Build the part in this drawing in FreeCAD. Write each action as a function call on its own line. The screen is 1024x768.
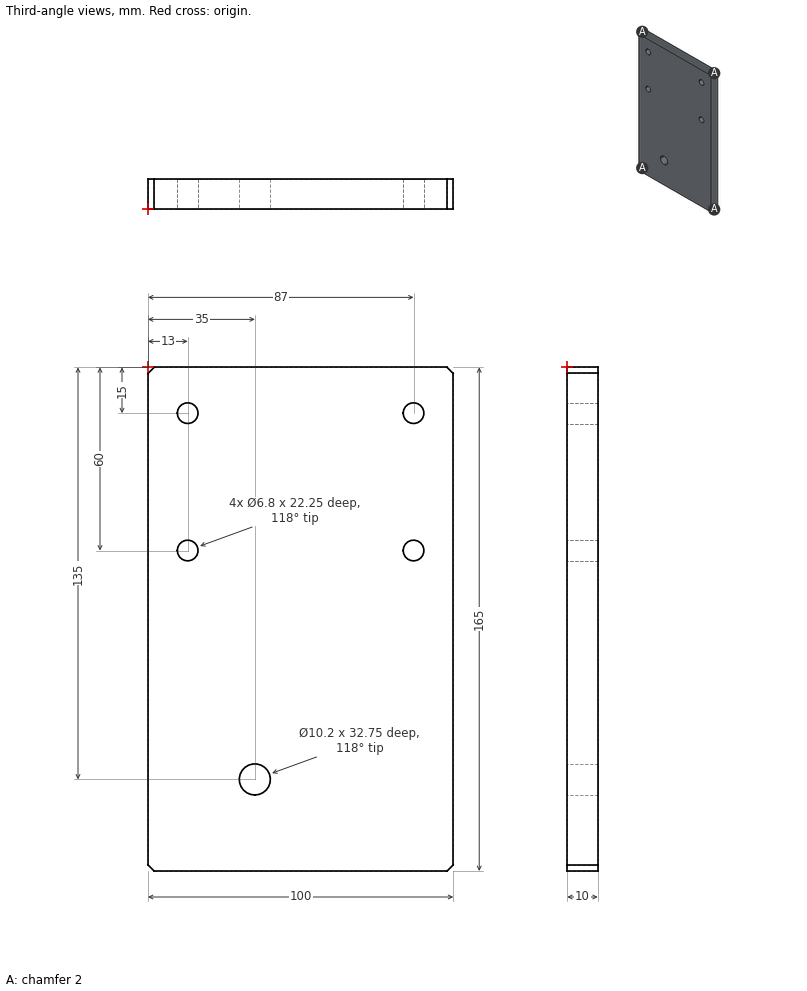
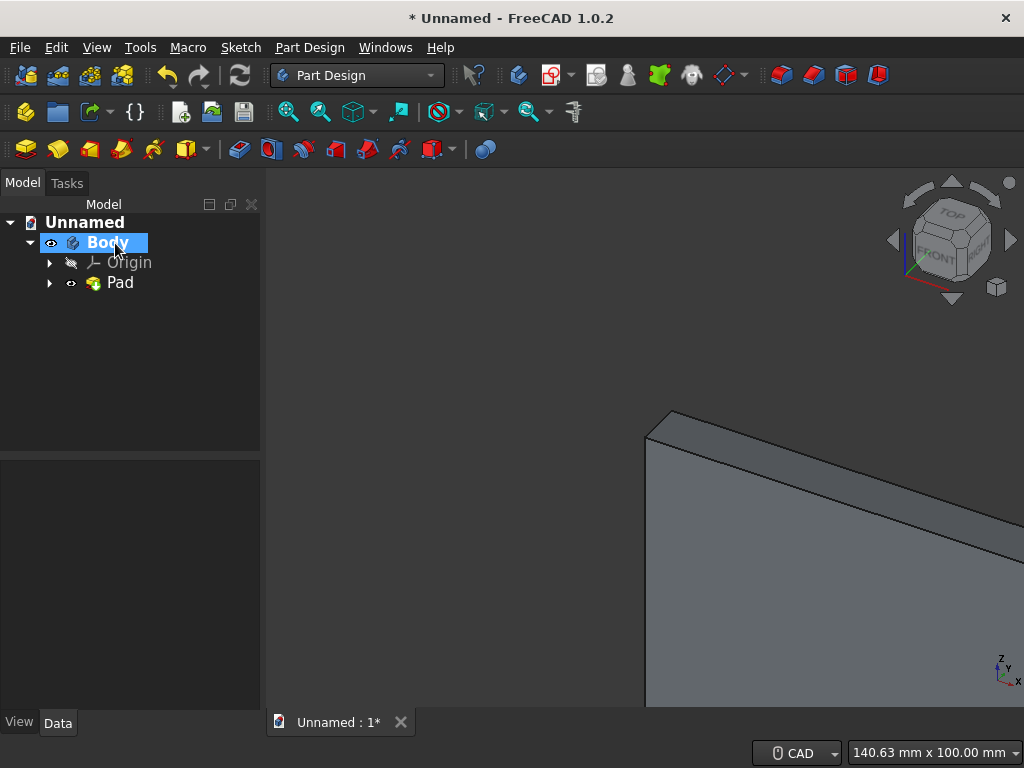
click(290, 112)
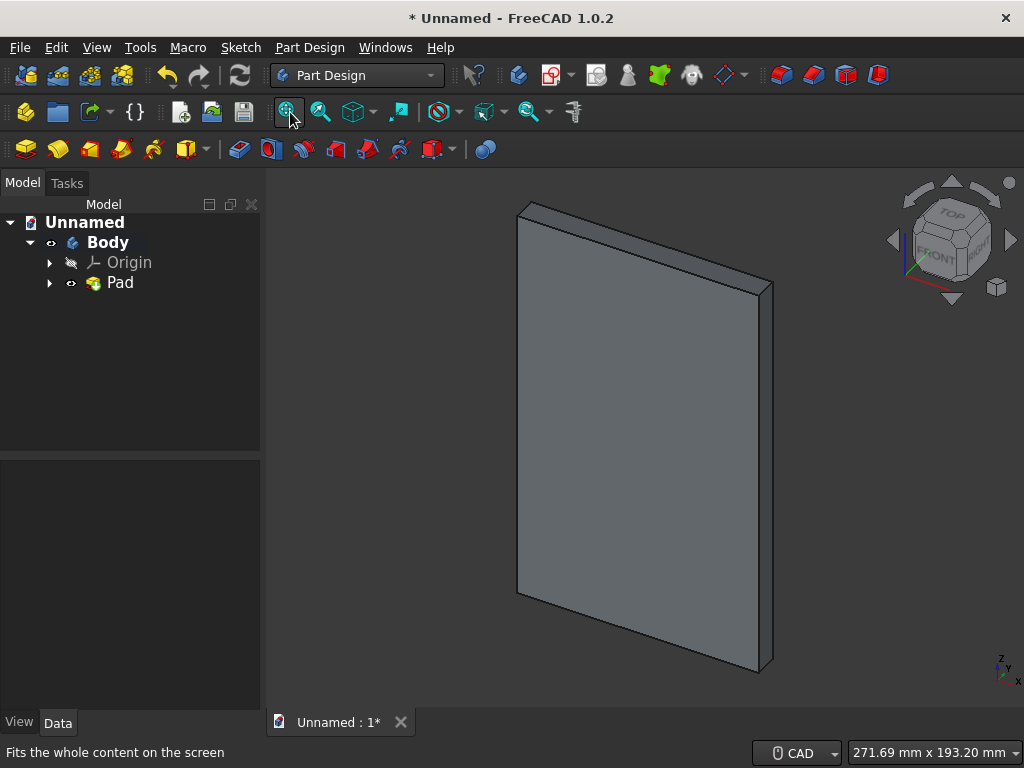
click(766, 288)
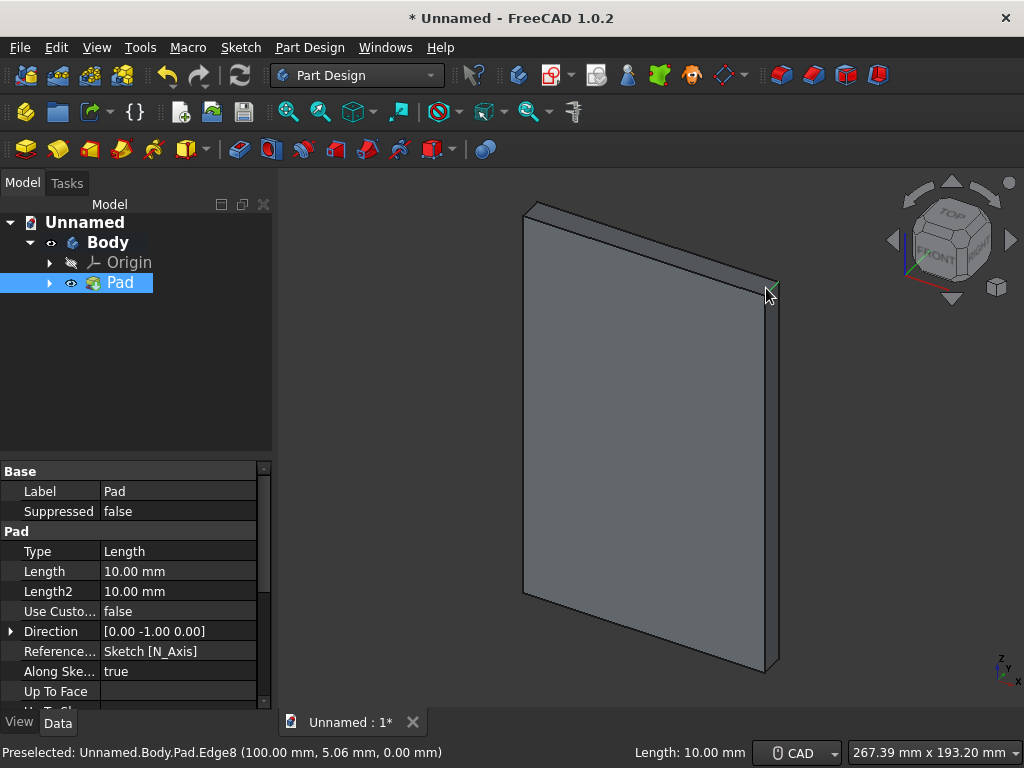
key(0)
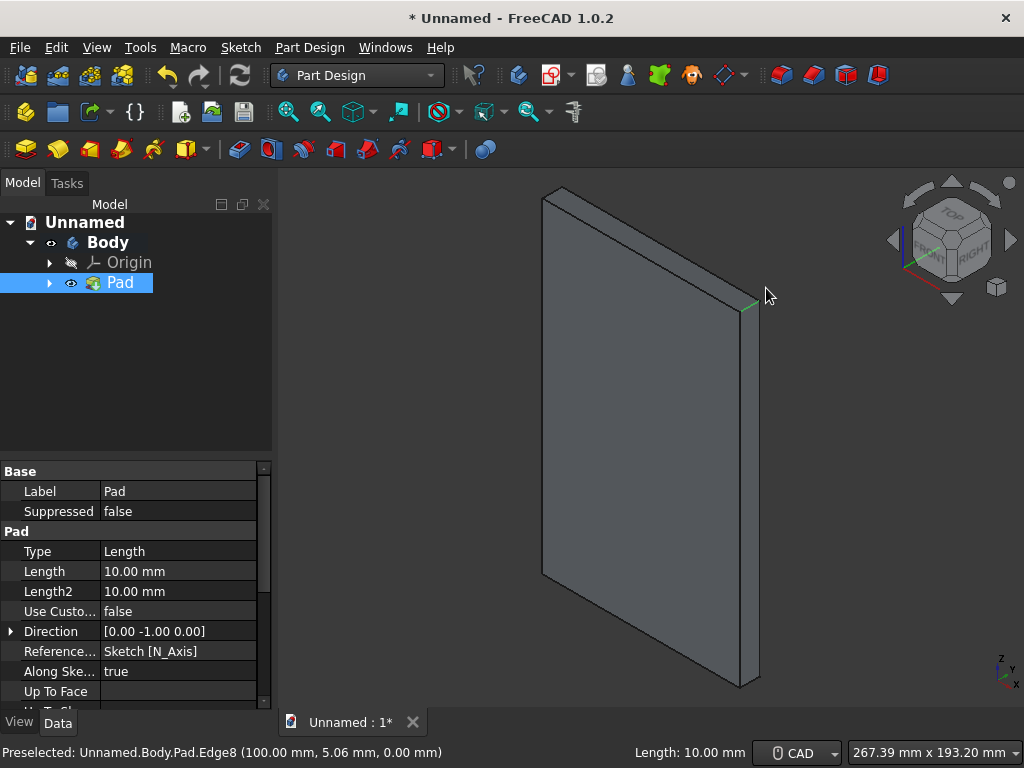
key(2)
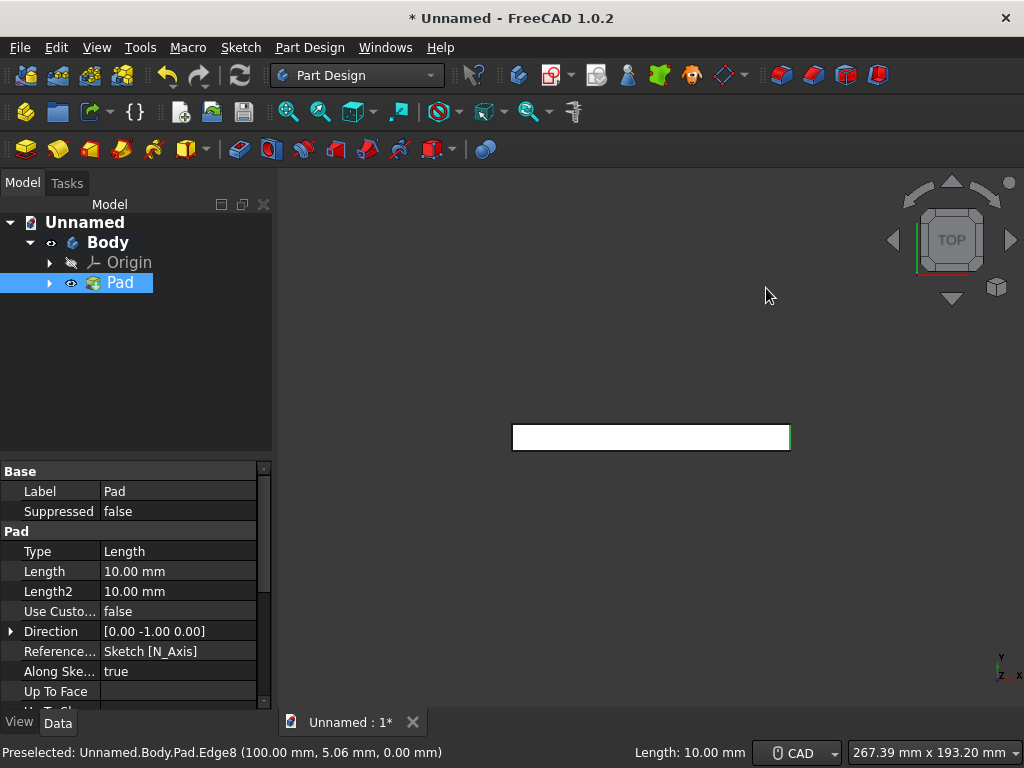
key(v)
key(f)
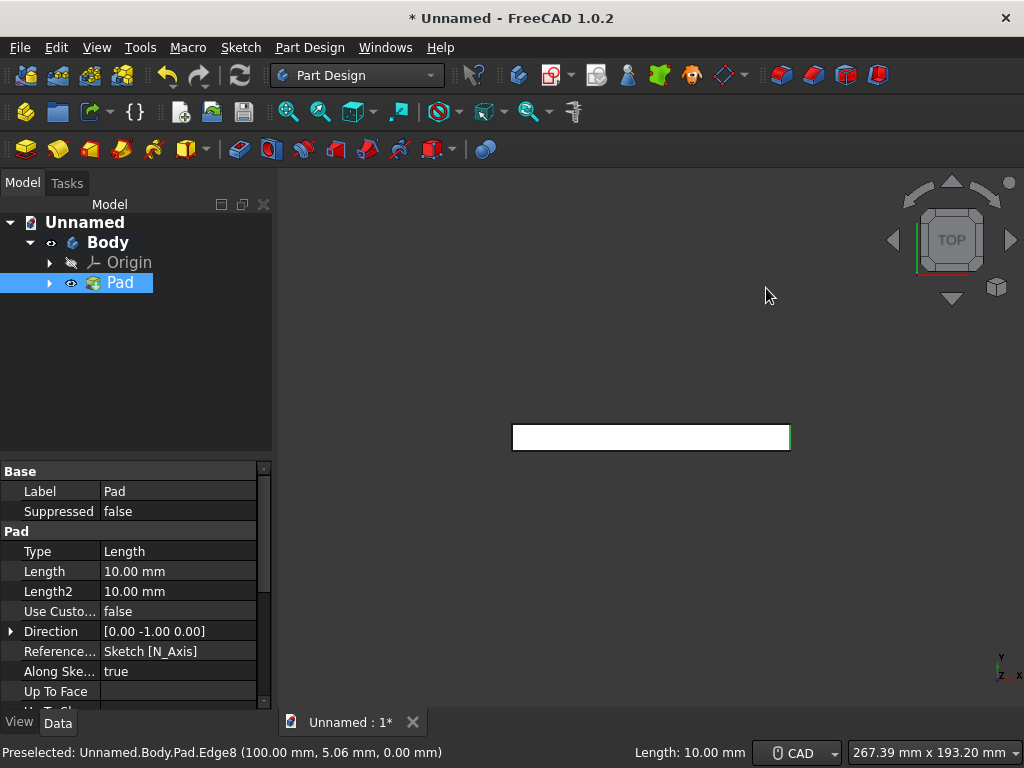
key(1)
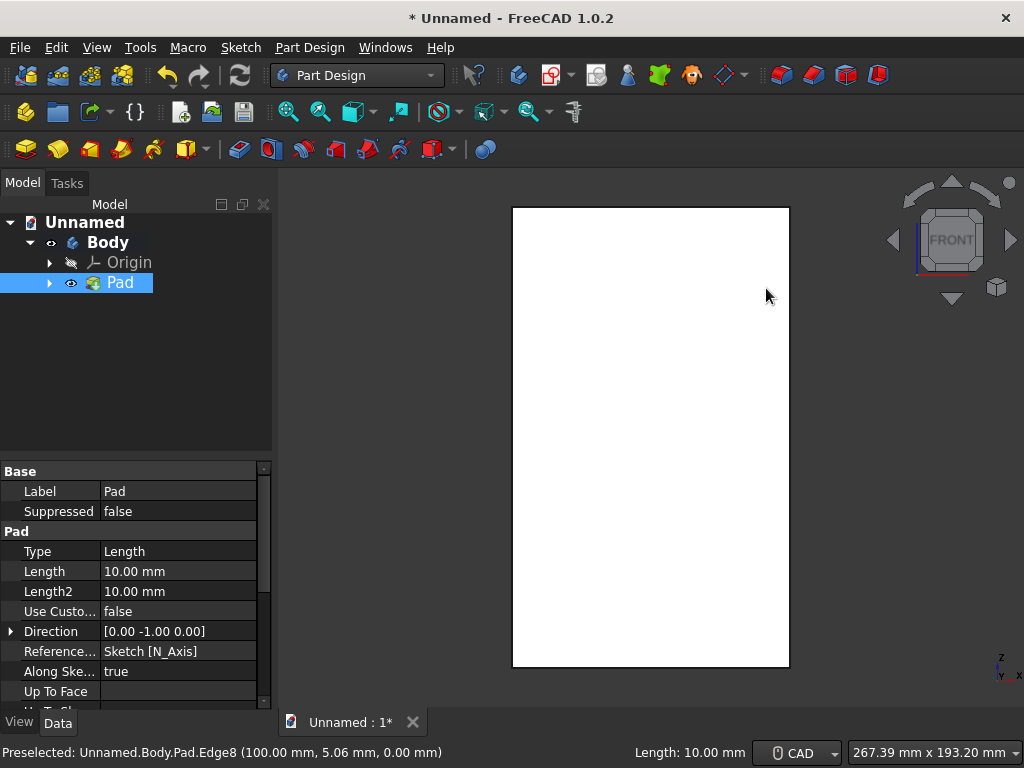
key(3)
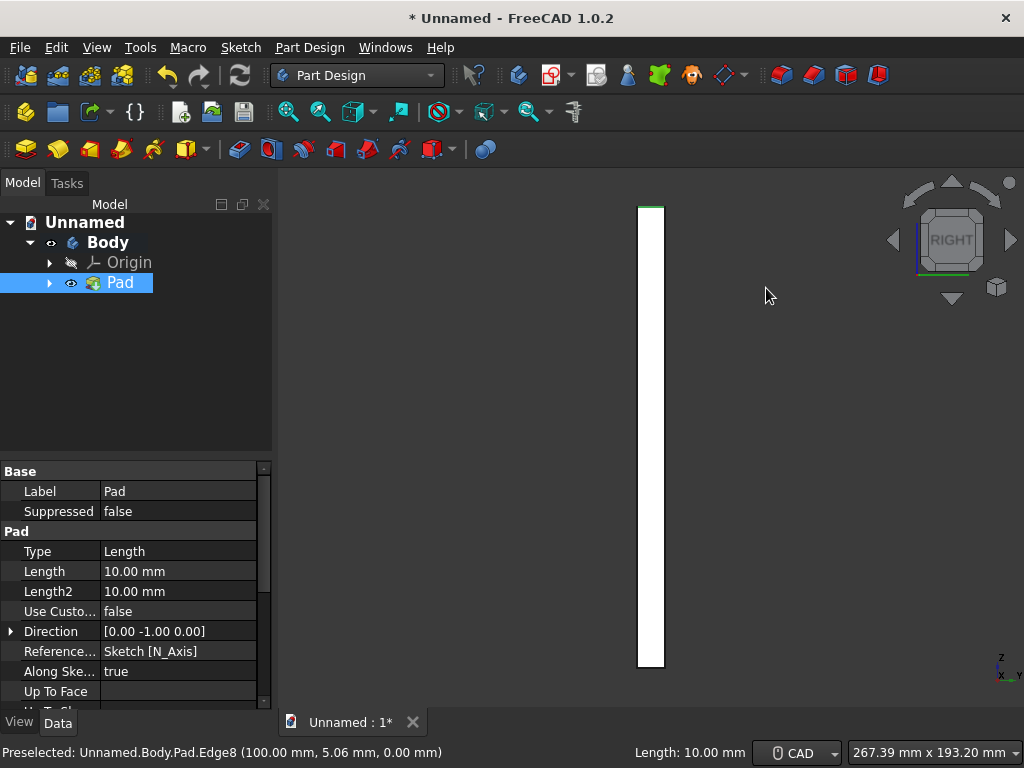
click(651, 667, ctrl)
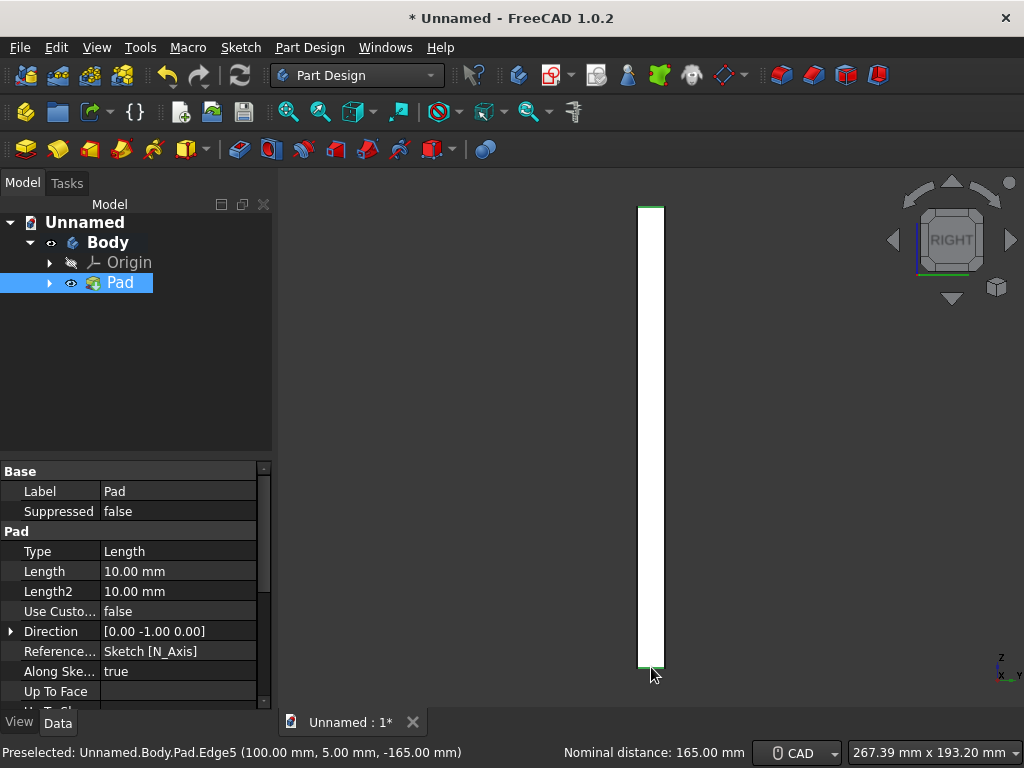
key(5)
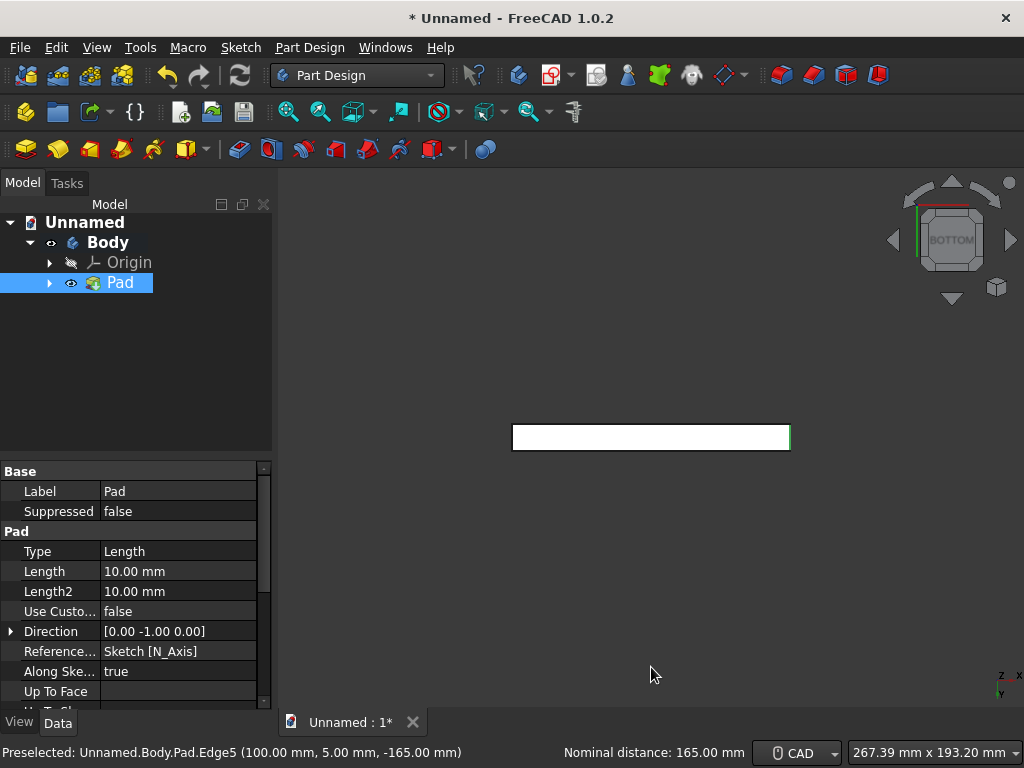
click(290, 112)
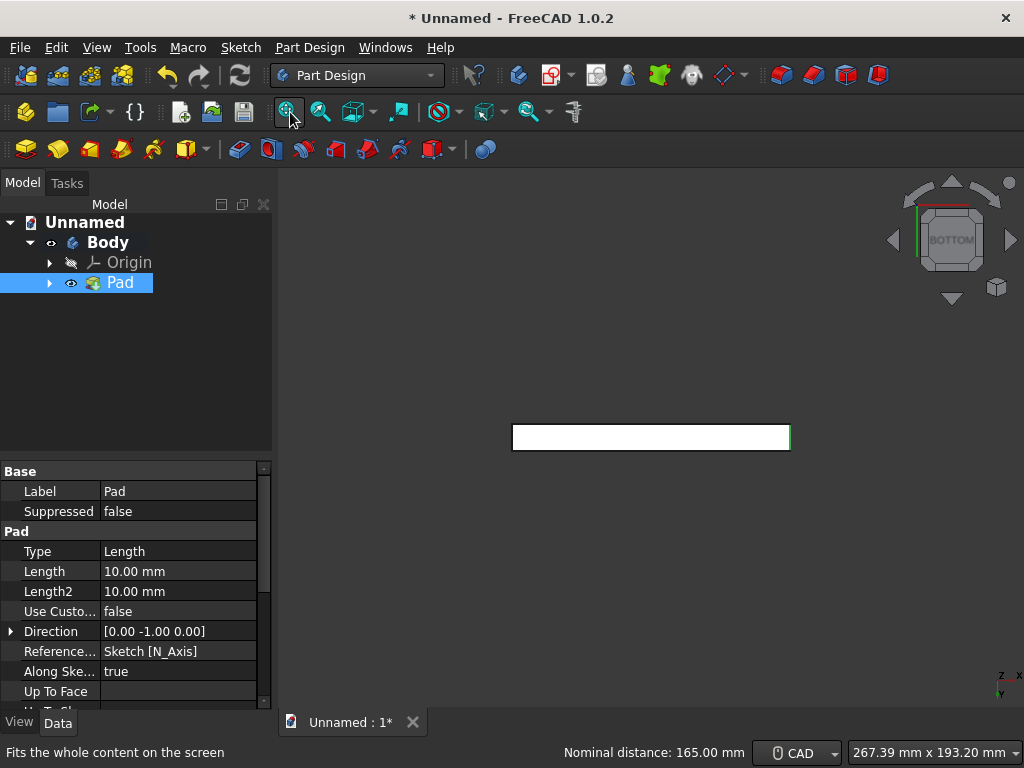
click(512, 436, ctrl)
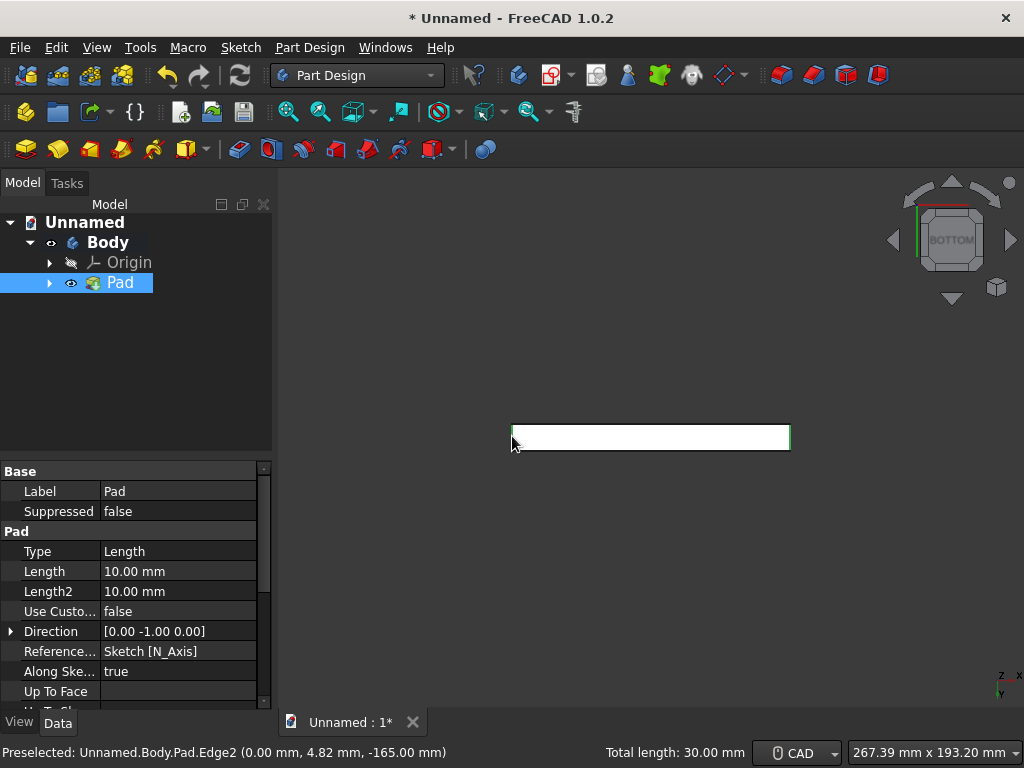
key(4)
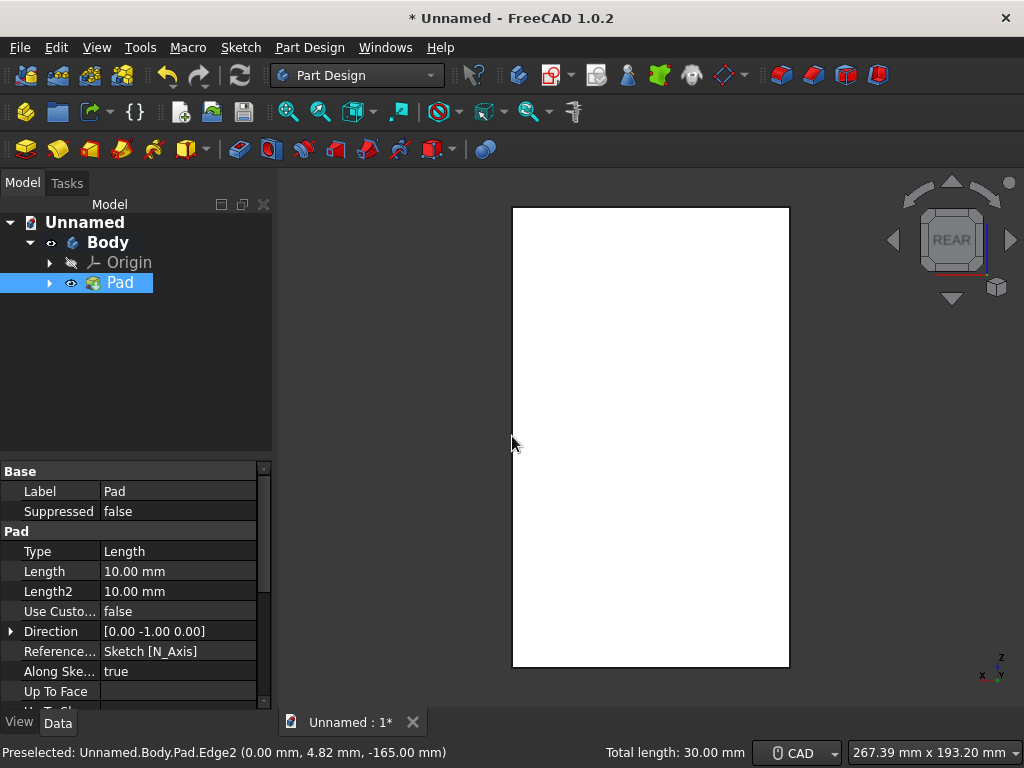
key(6)